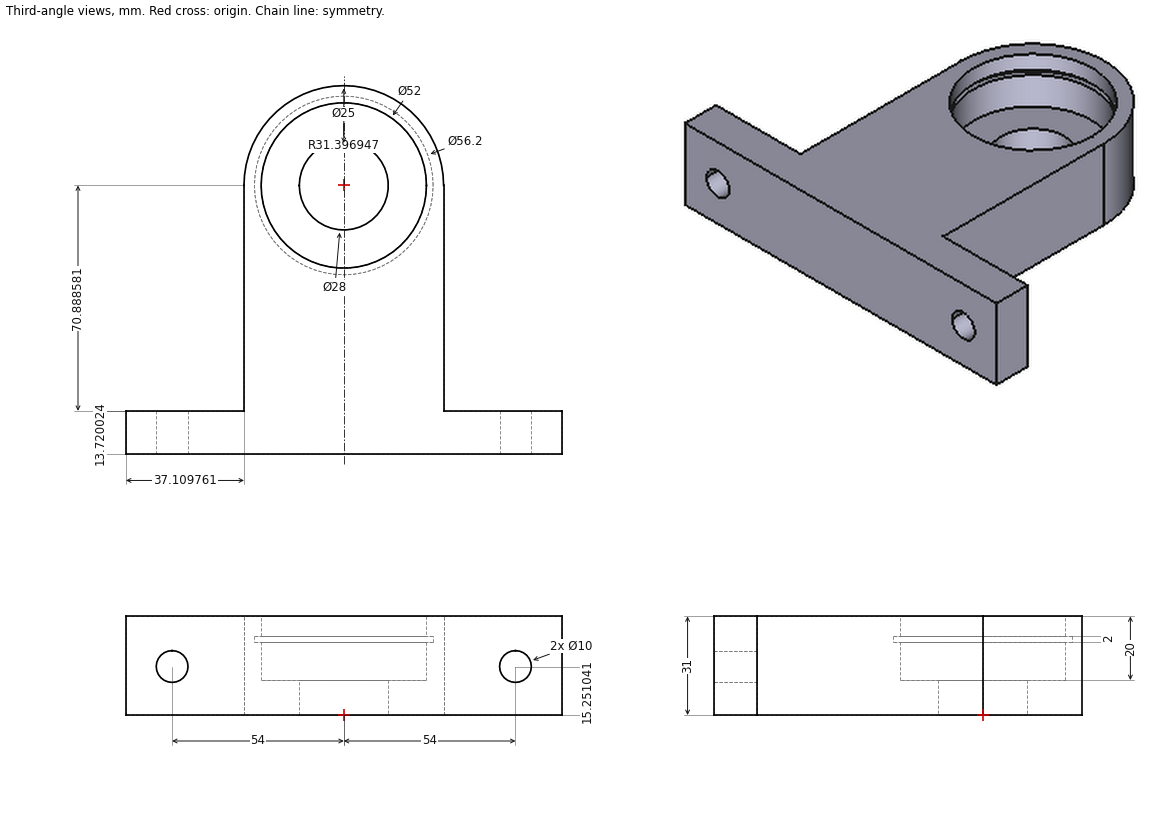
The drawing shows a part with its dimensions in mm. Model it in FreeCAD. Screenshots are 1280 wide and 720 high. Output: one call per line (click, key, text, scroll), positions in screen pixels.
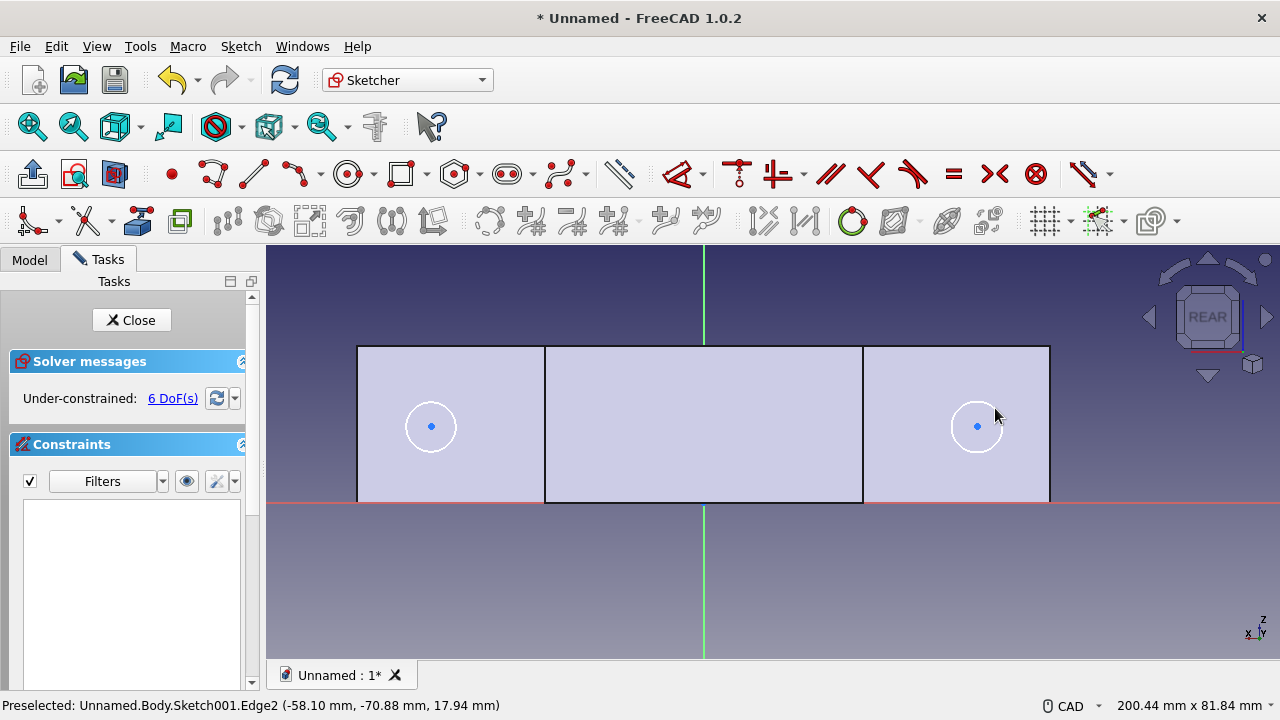
click(448, 409)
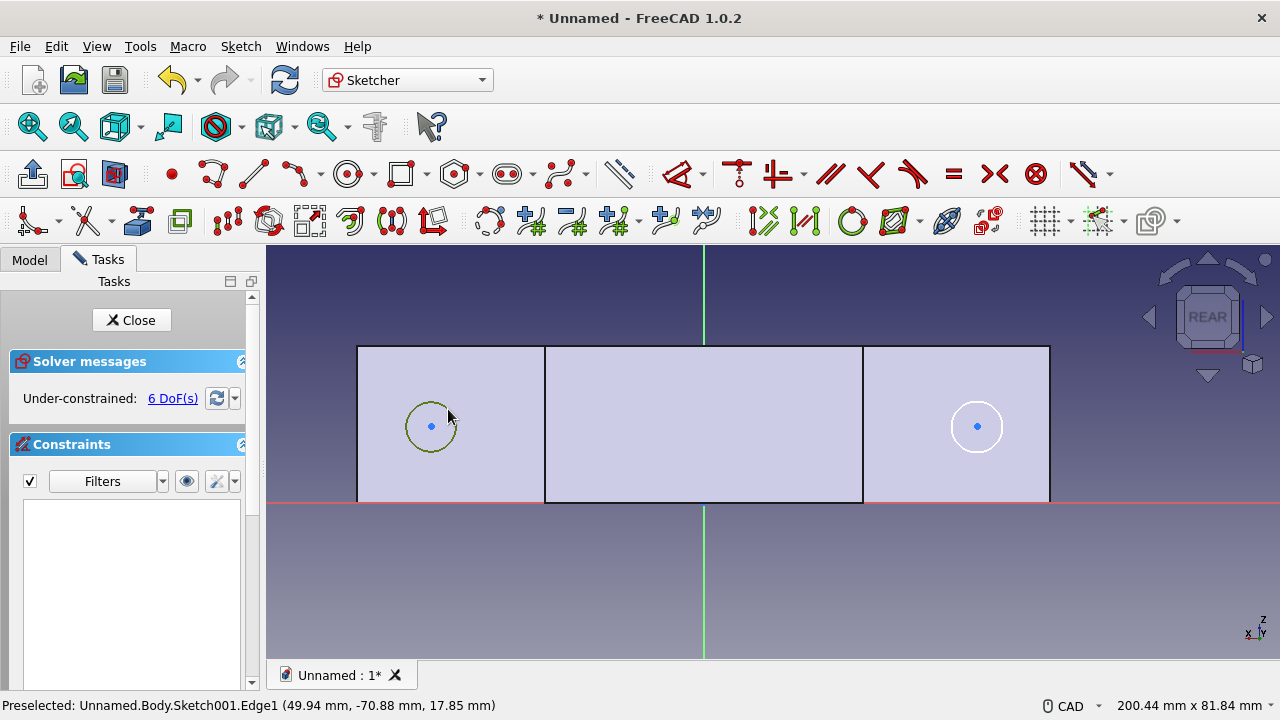
click(995, 409)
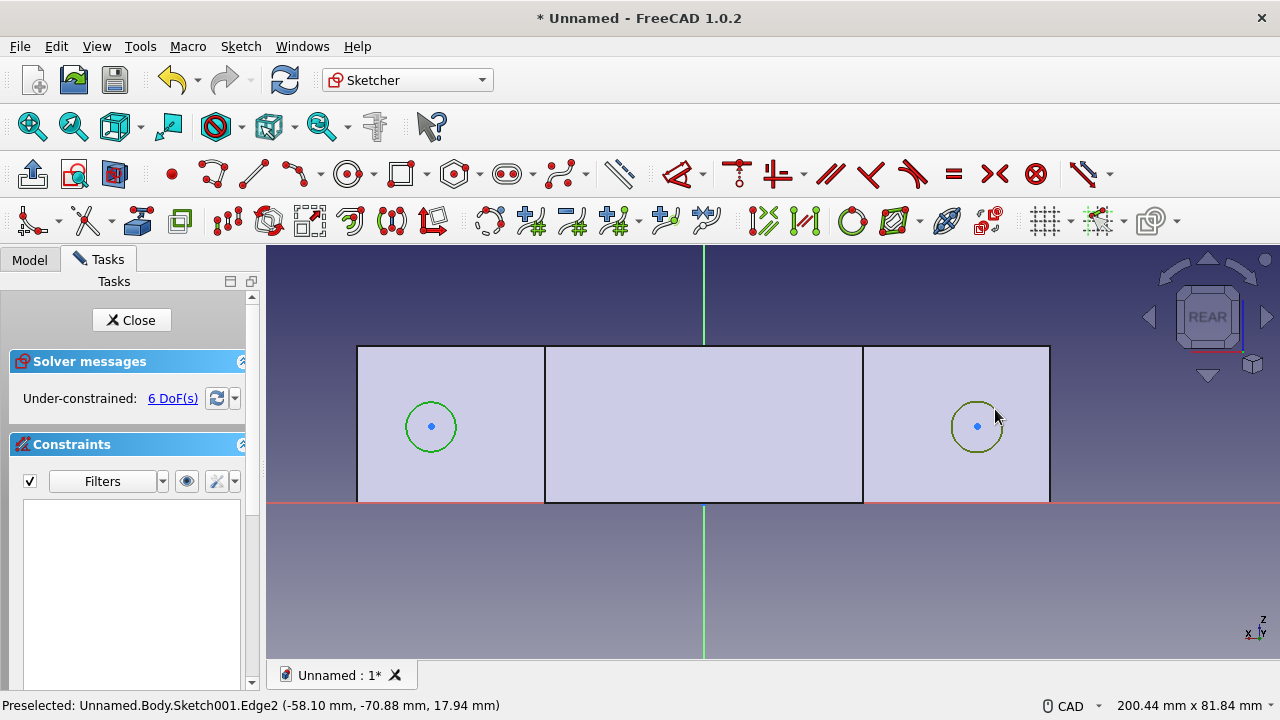
click(954, 174)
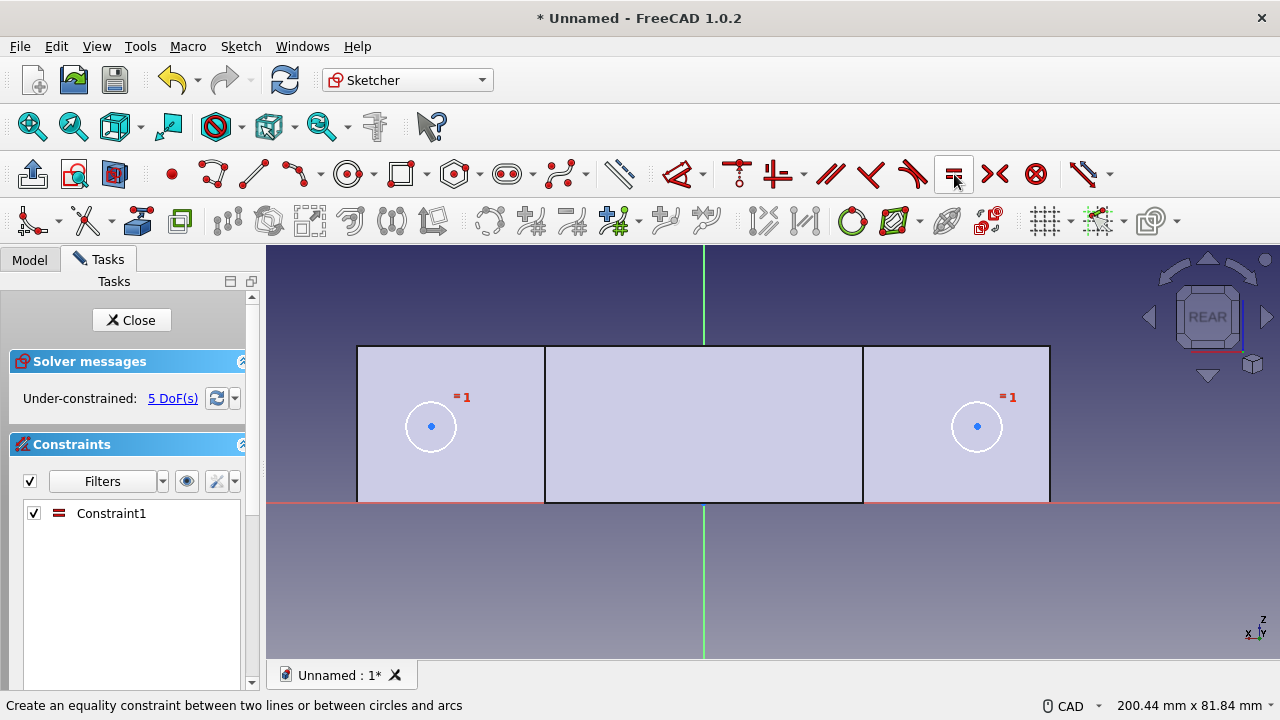
click(431, 427)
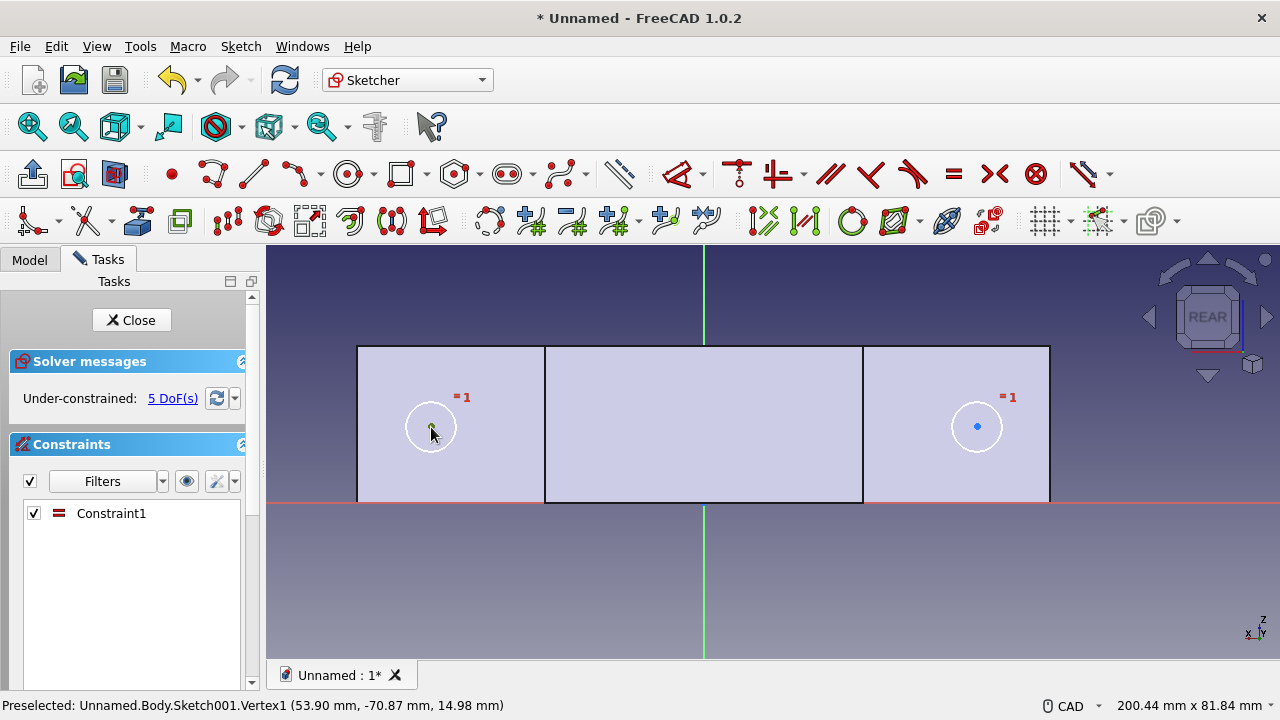
click(977, 427)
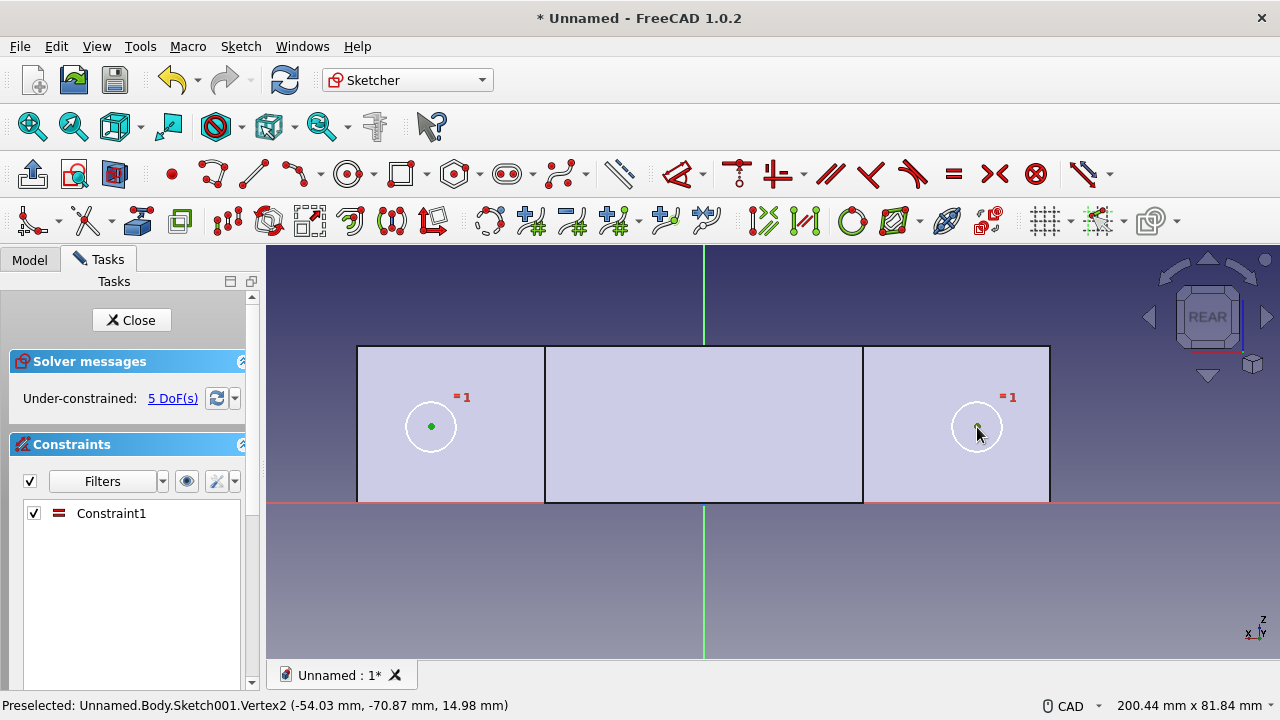
click(804, 174)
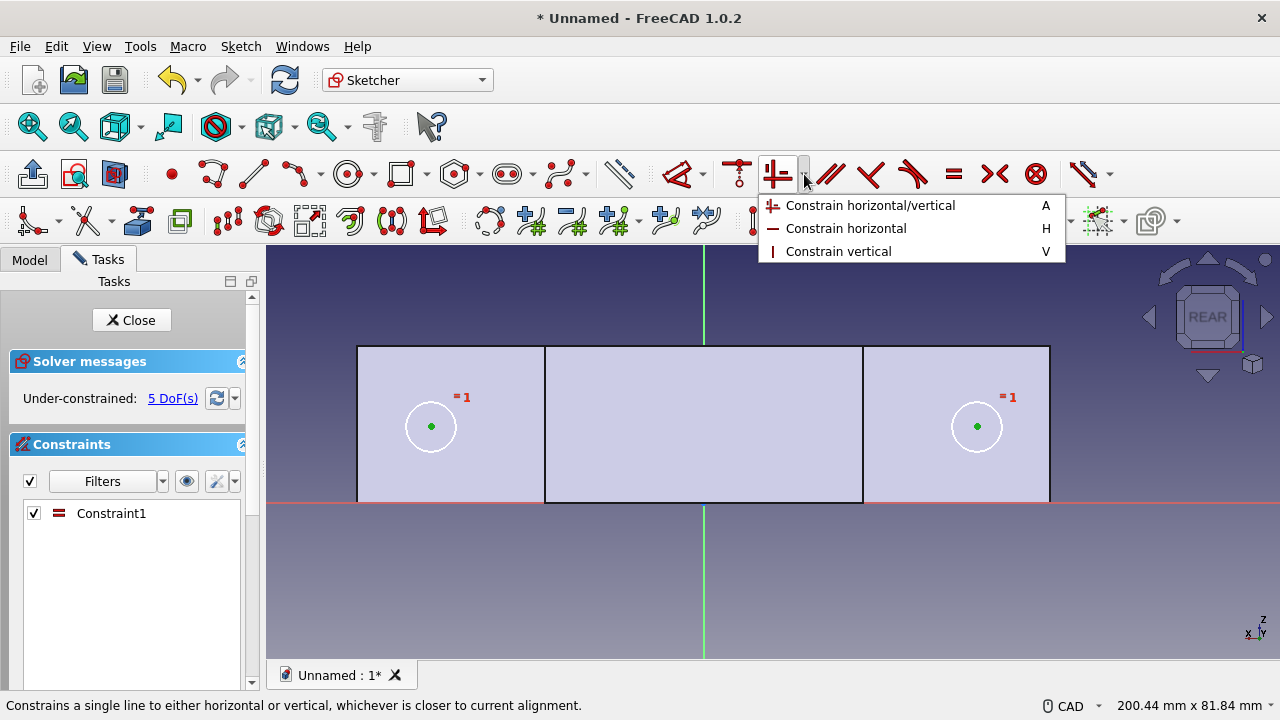
click(912, 228)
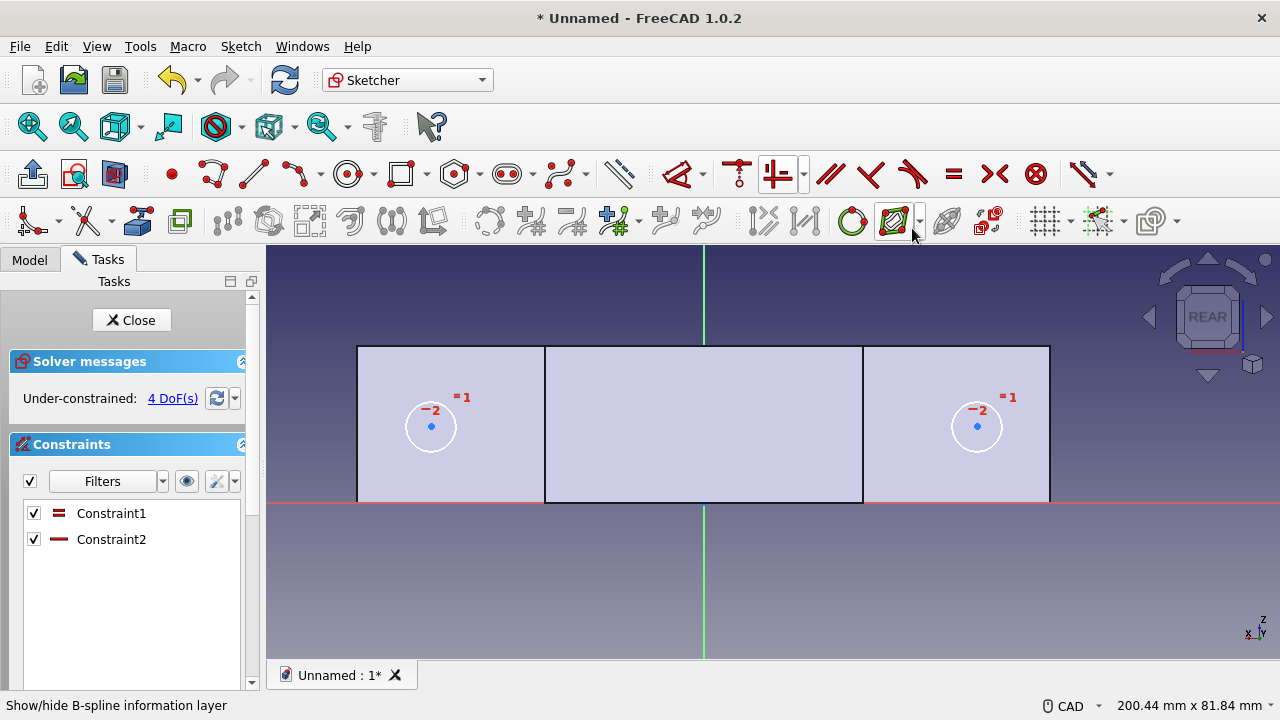
click(676, 174)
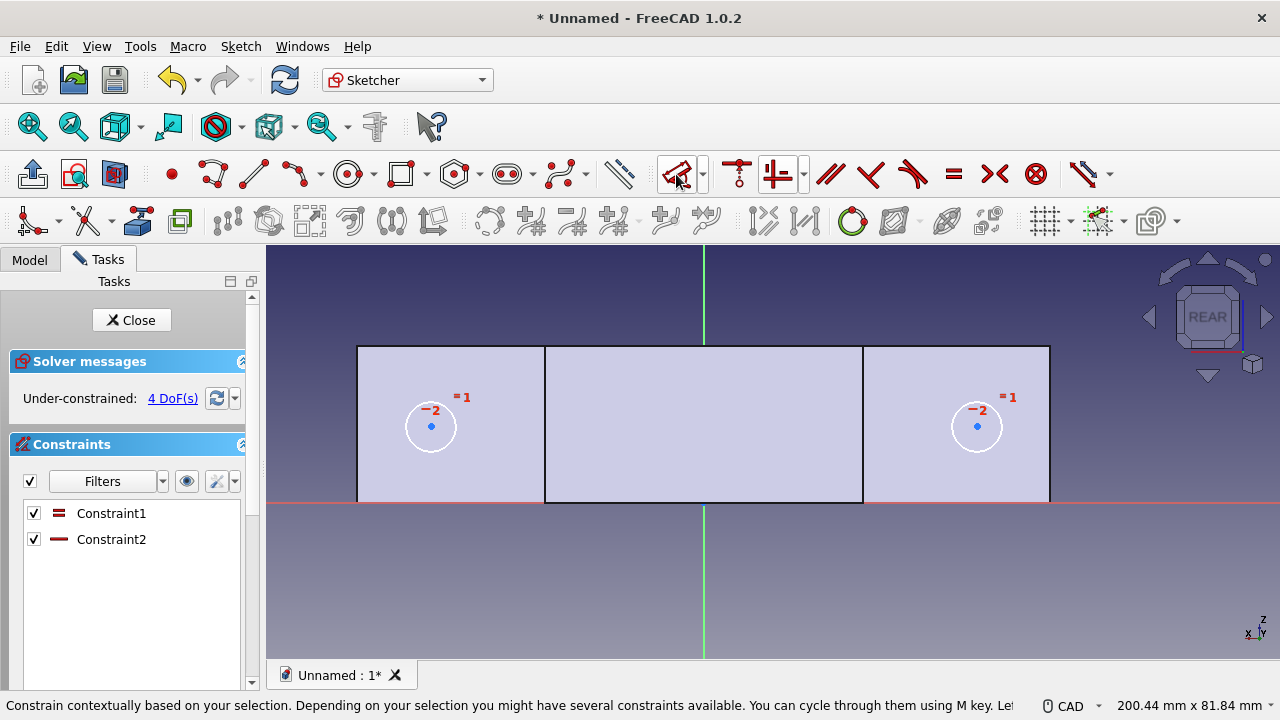
click(448, 409)
click(470, 386)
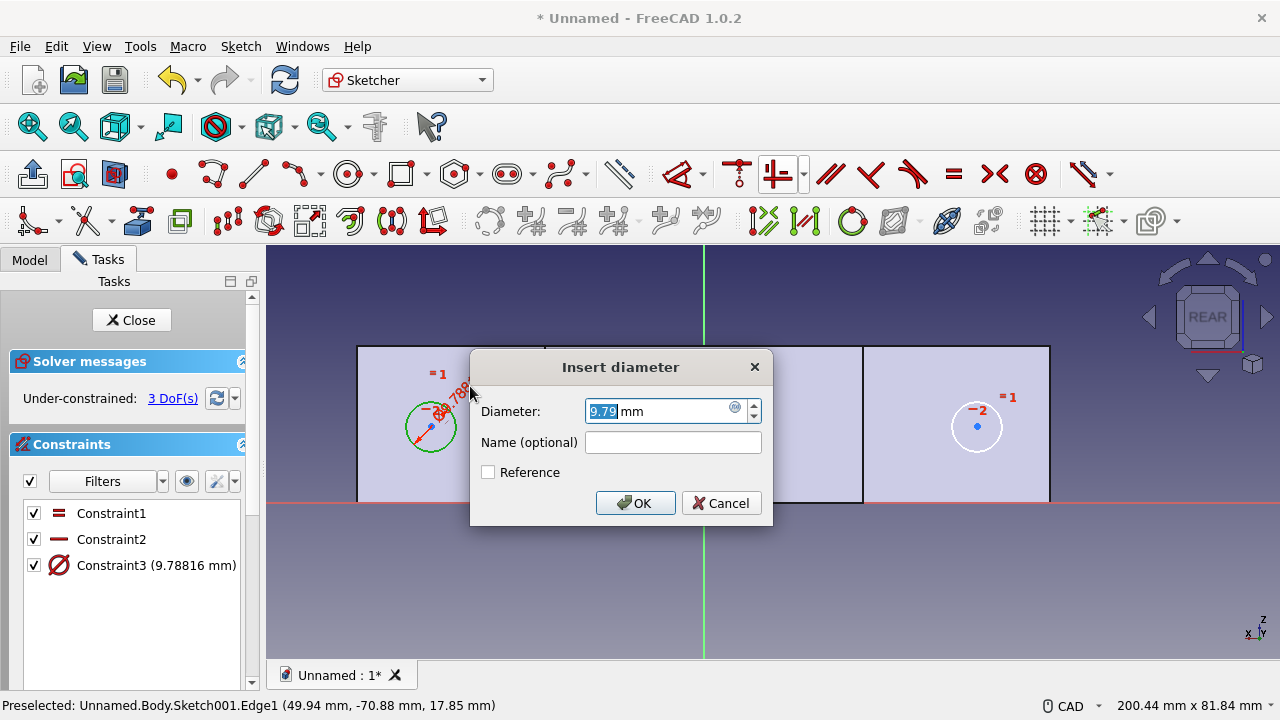
text(10)
key(Return)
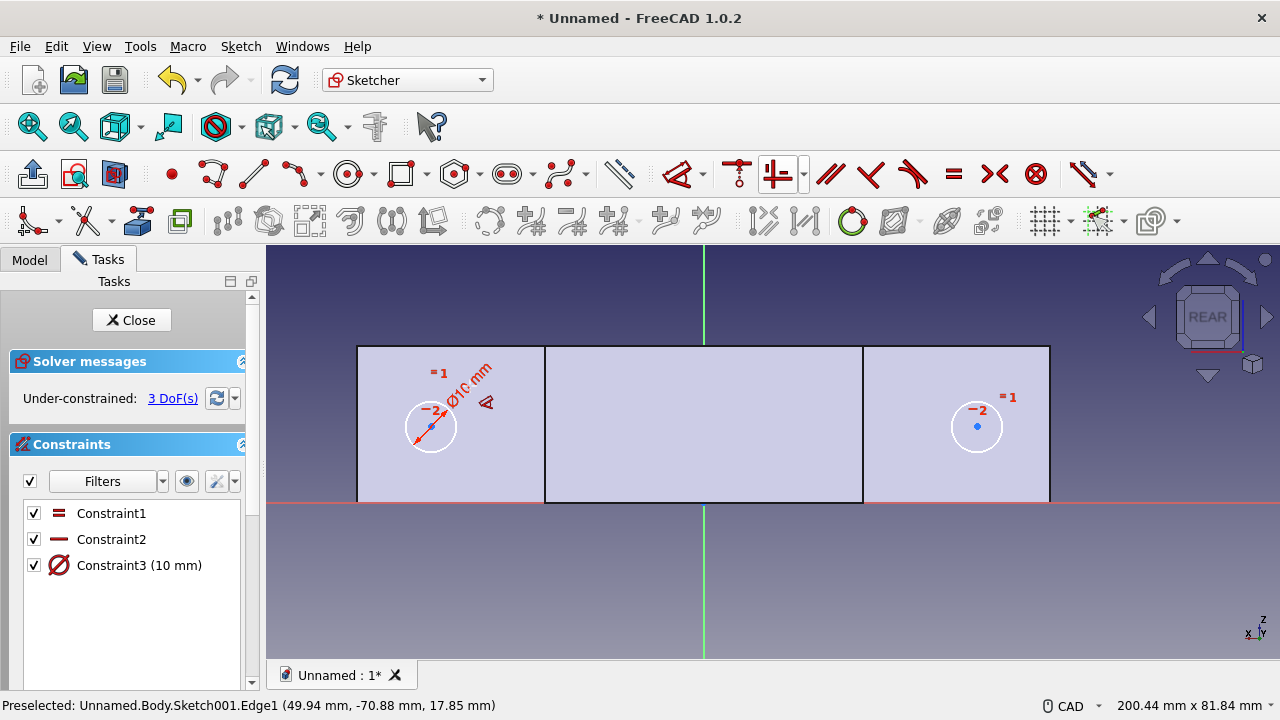
click(431, 427)
click(567, 537)